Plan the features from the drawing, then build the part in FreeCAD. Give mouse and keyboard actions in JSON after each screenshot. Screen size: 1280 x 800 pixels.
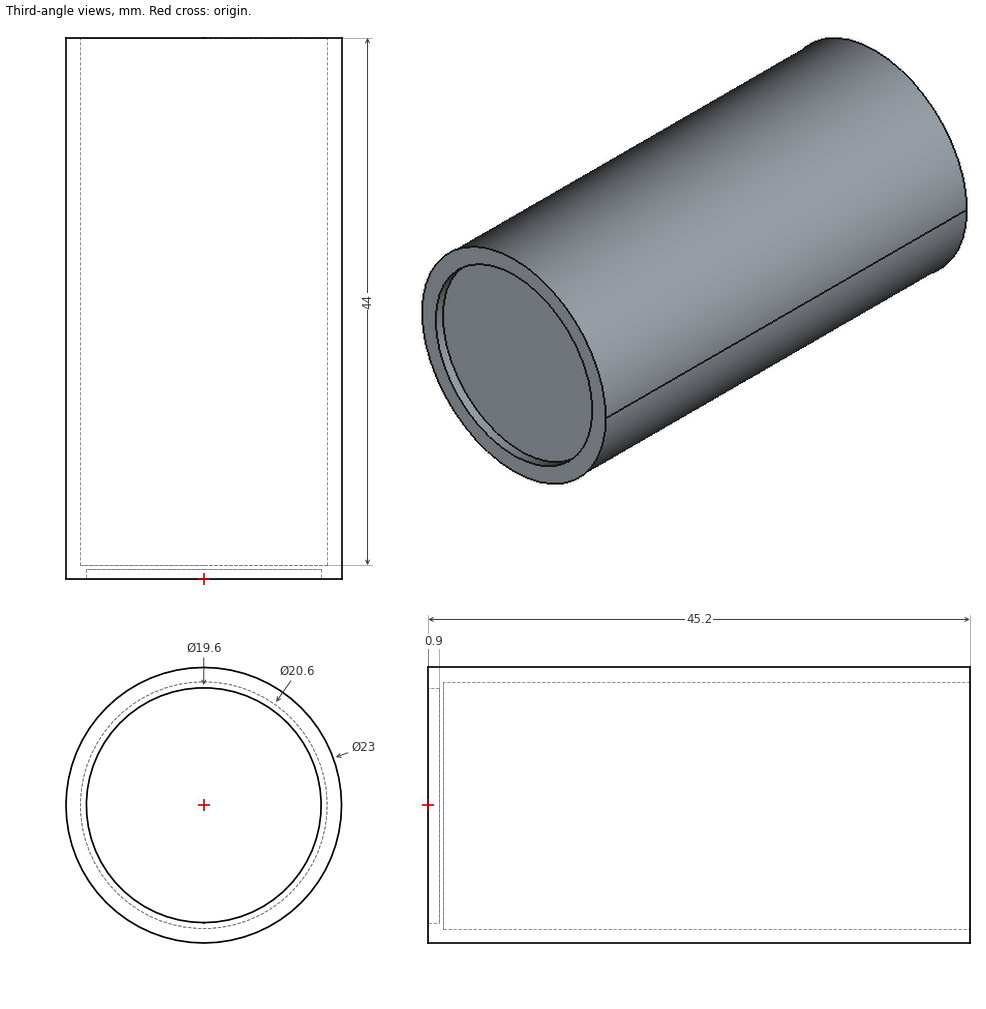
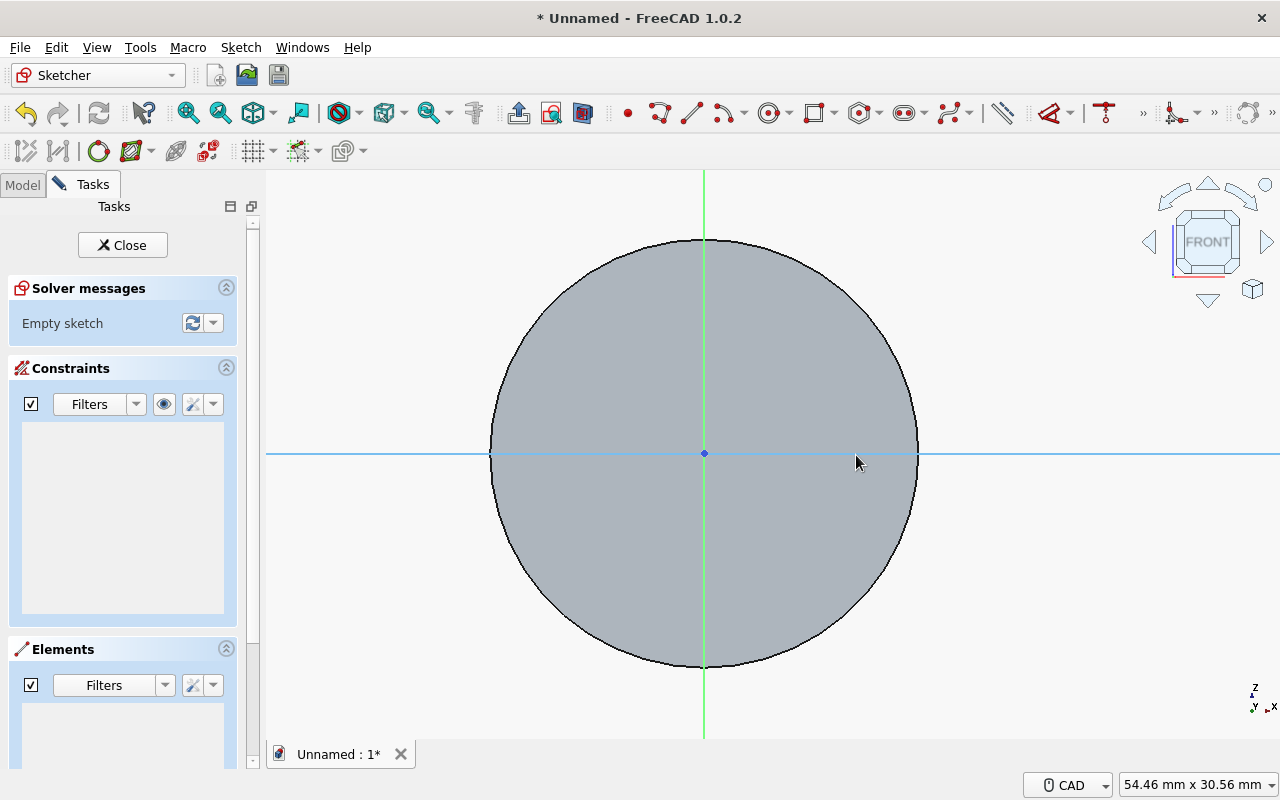
{"action": "left_click", "coordinate": [770, 114]}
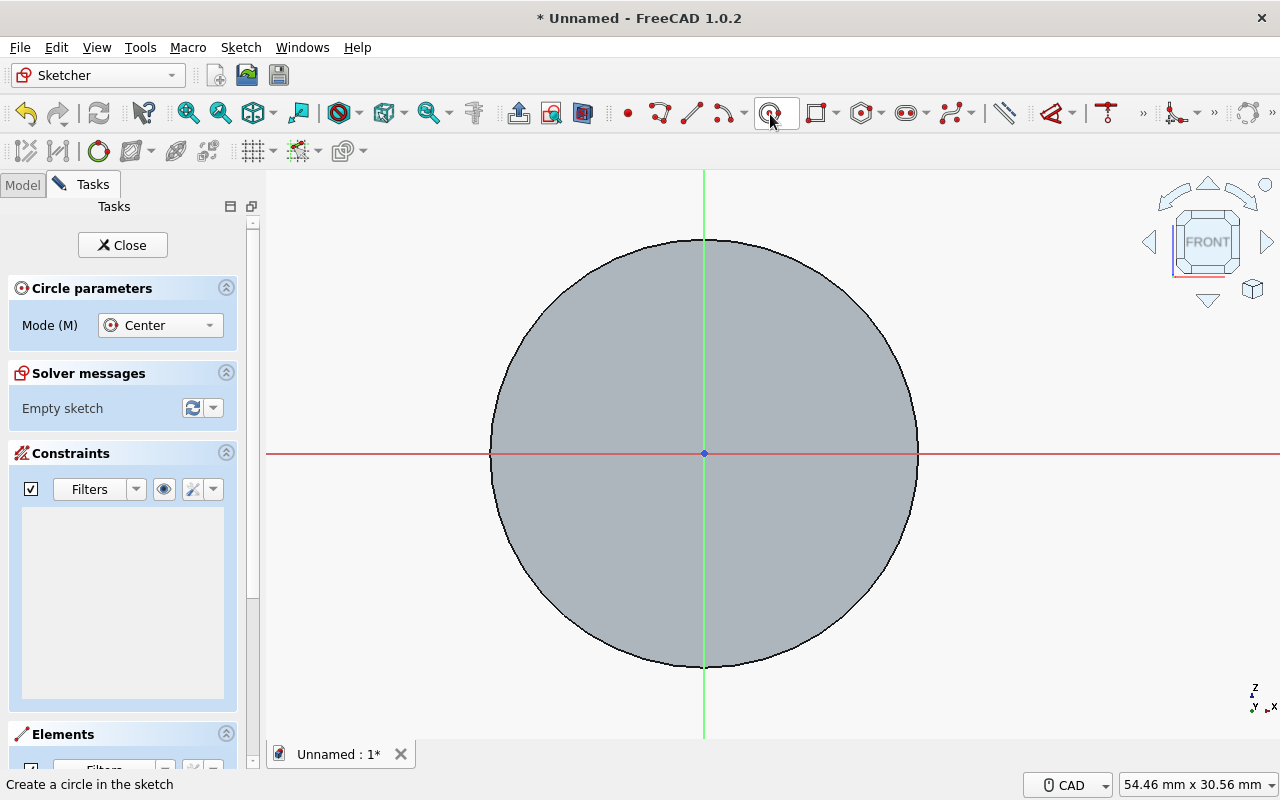
{"action": "left_click", "coordinate": [704, 454]}
{"action": "mouse_move", "coordinate": [833, 325]}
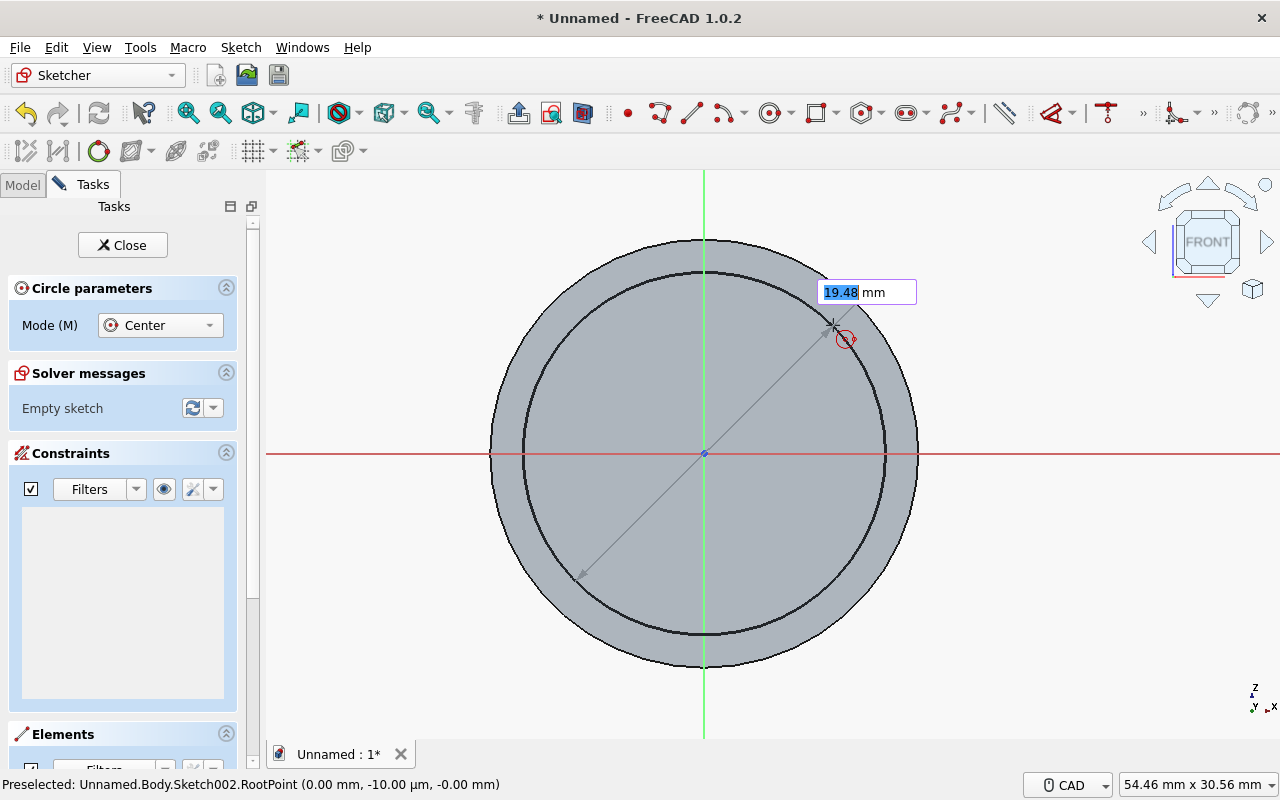
{"action": "type", "text": "19.6"}
{"action": "key", "text": "Return"}
{"action": "key", "text": "Escape"}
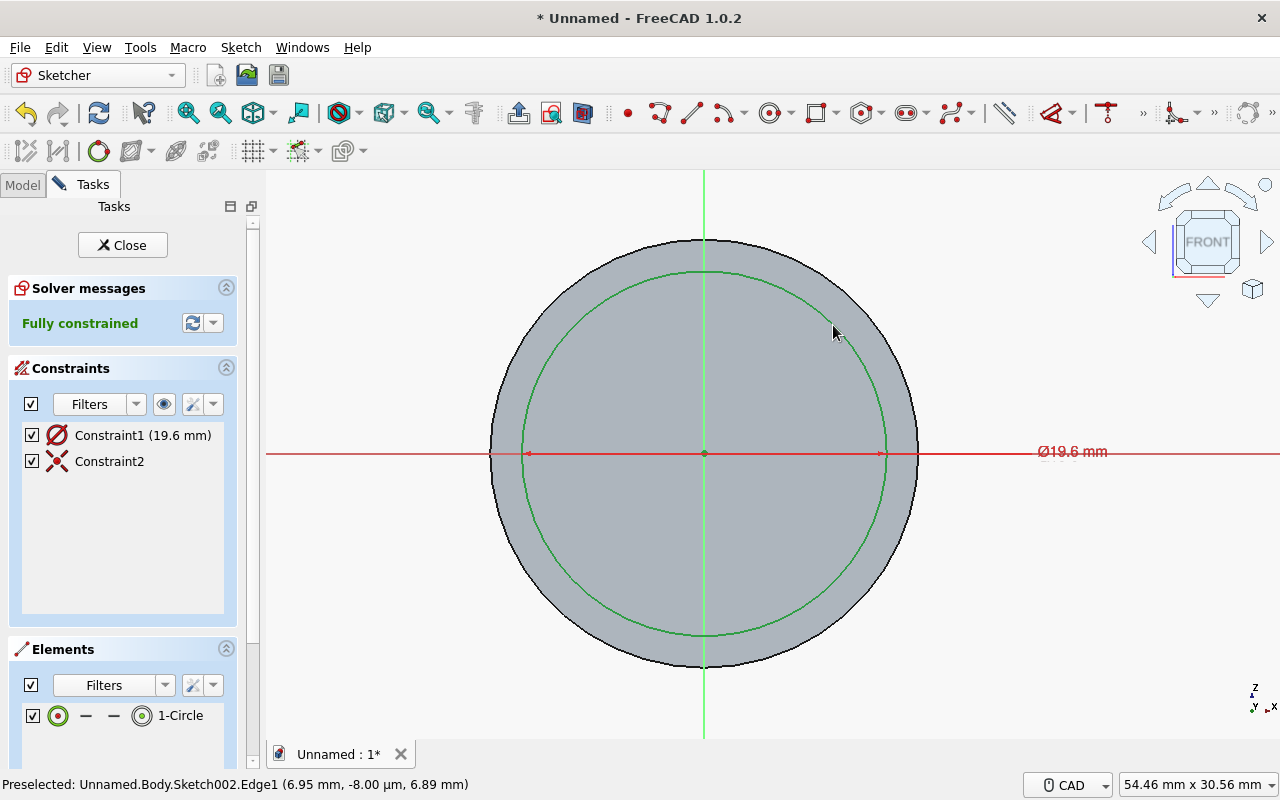
{"action": "left_click", "coordinate": [123, 245]}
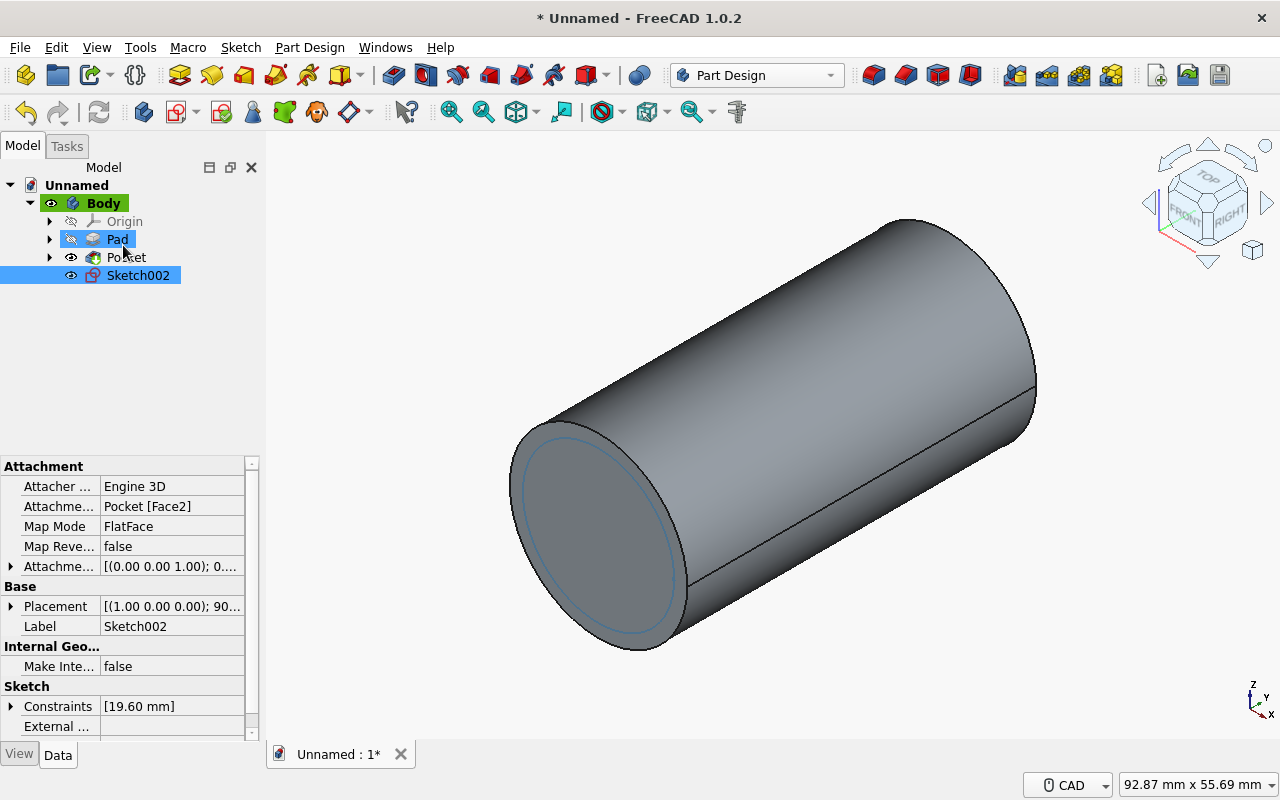
{"action": "left_click", "coordinate": [394, 76]}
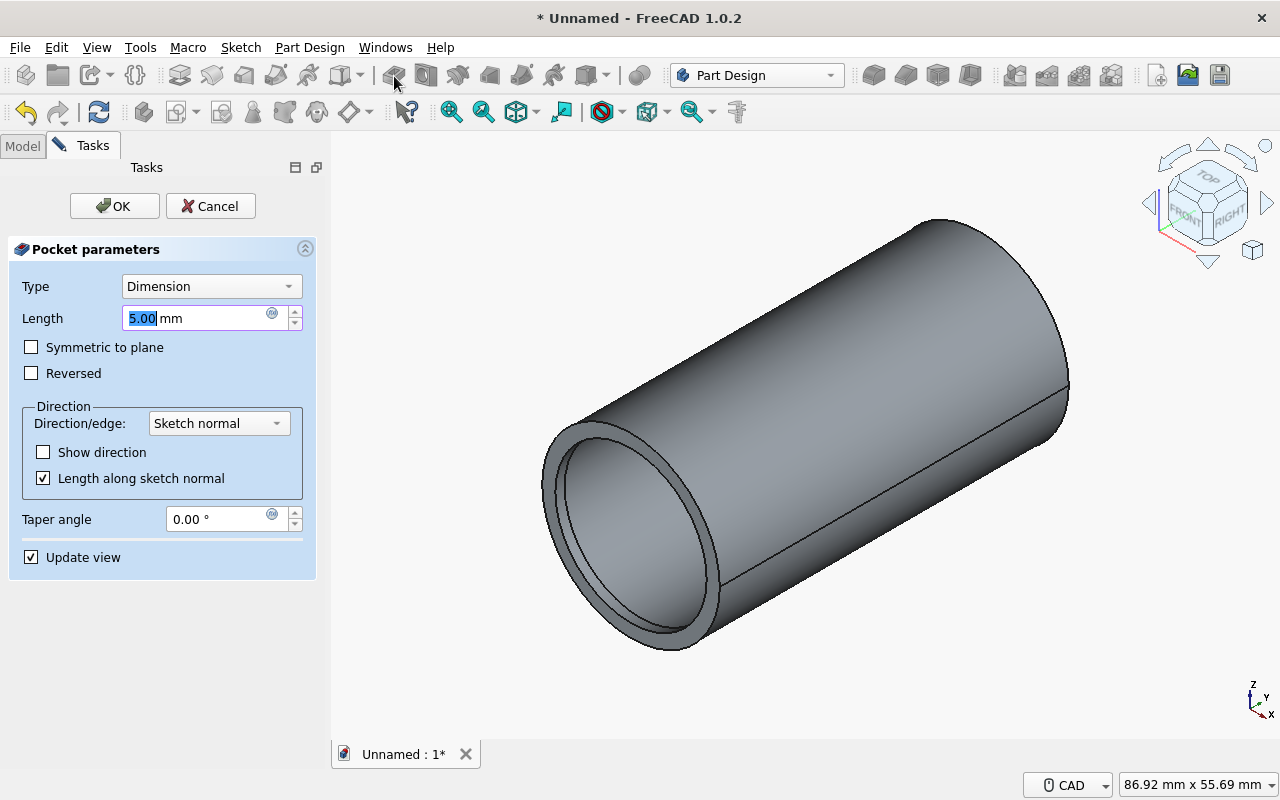
{"action": "type", "text": "0.9"}
{"action": "key", "text": "Tab"}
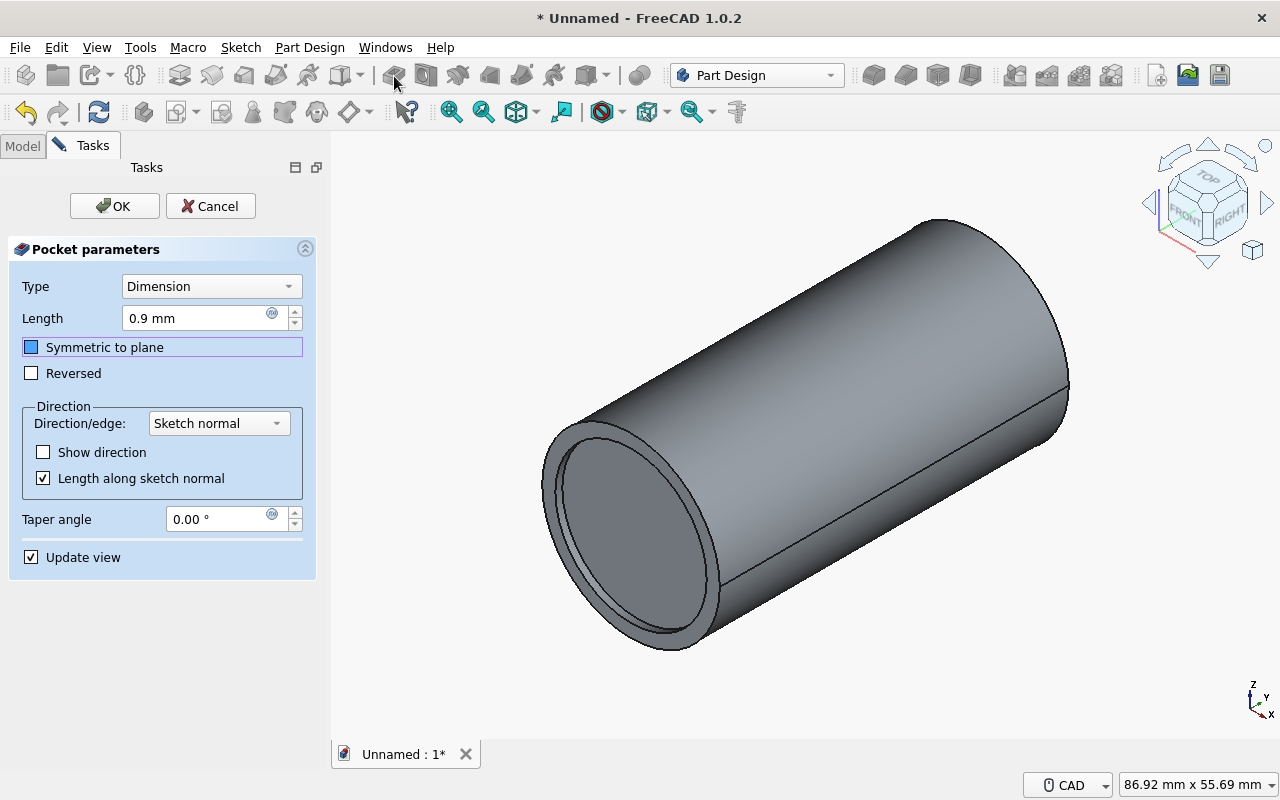
{"action": "left_click", "coordinate": [115, 206]}